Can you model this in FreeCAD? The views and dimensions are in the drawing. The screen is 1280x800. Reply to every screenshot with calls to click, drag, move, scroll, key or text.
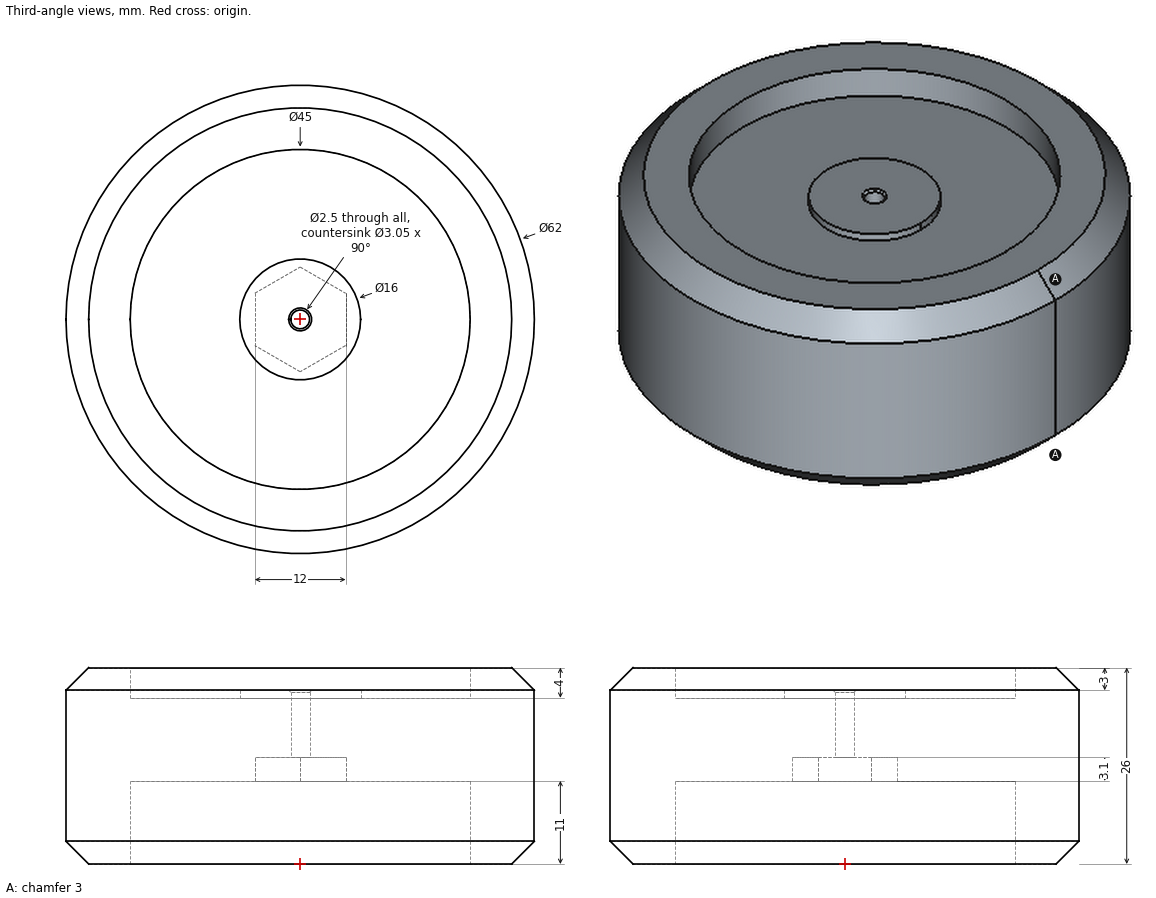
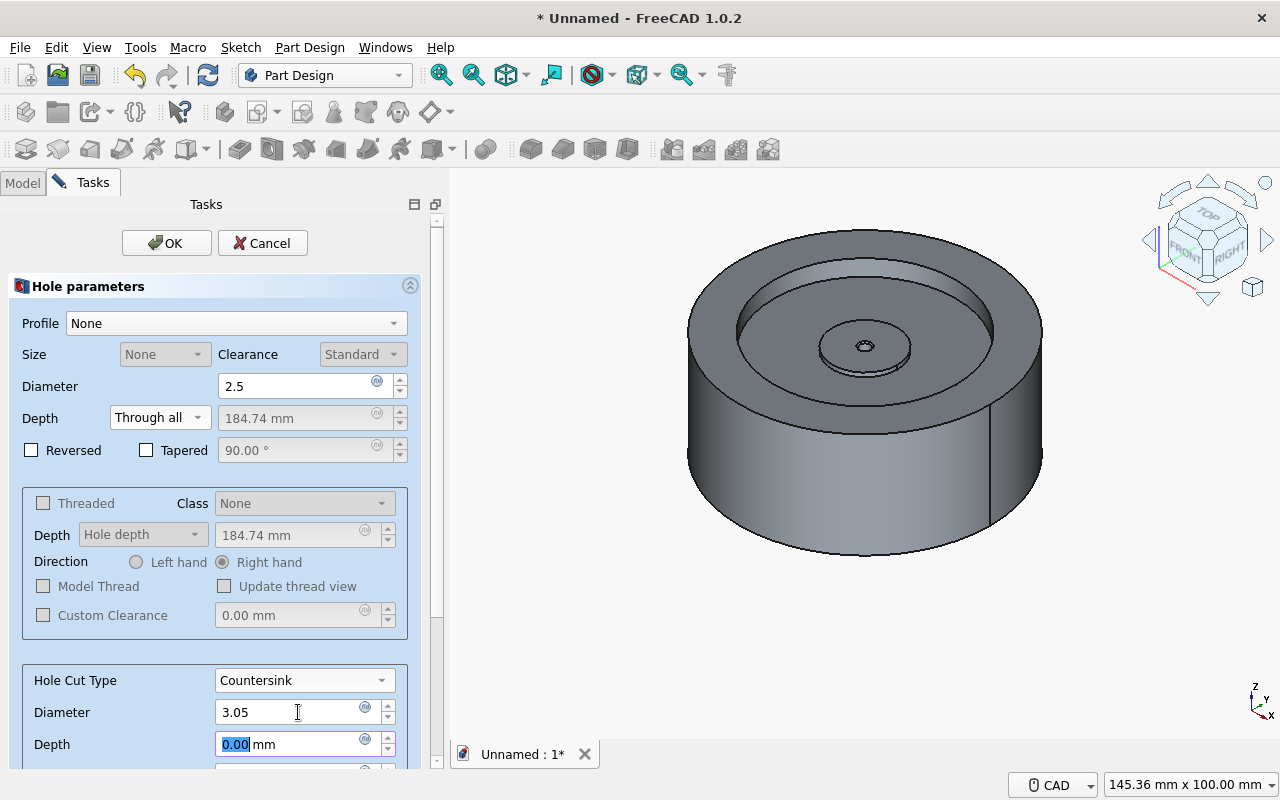
click(167, 243)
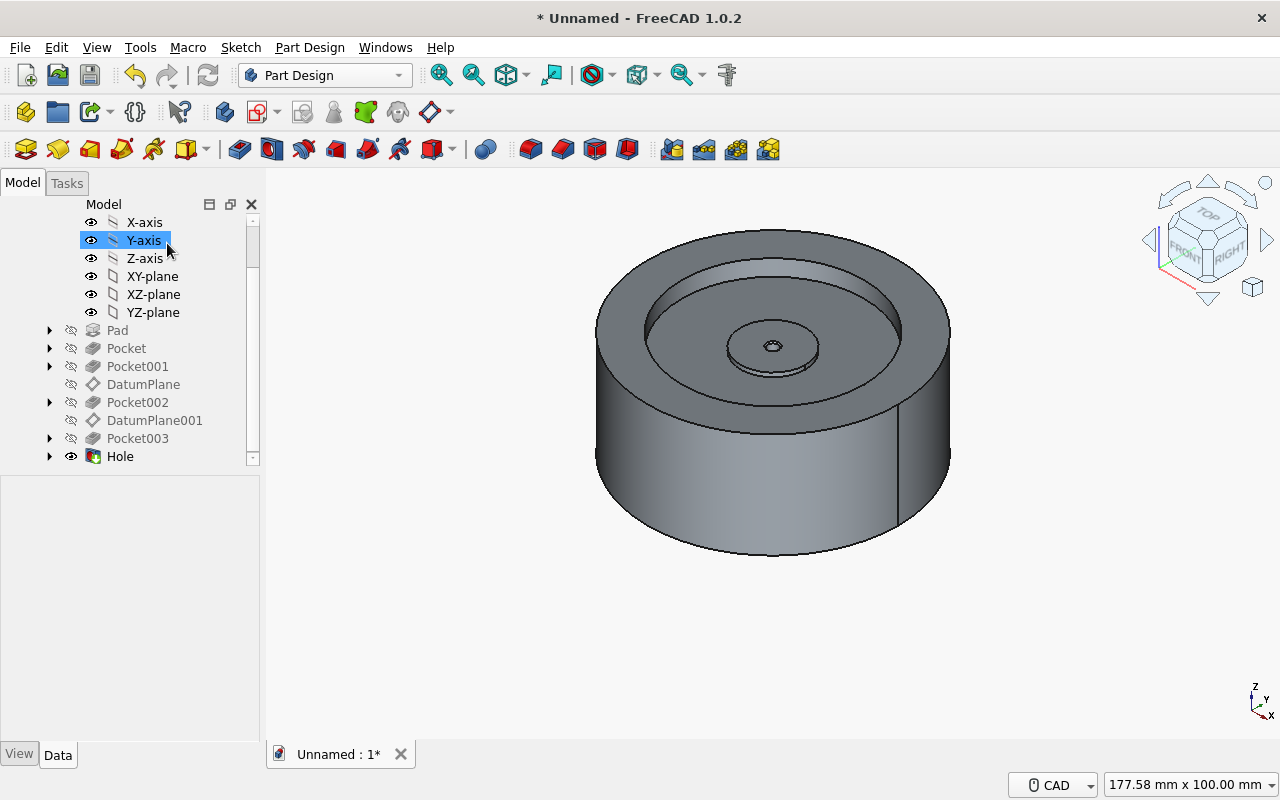
click(693, 544)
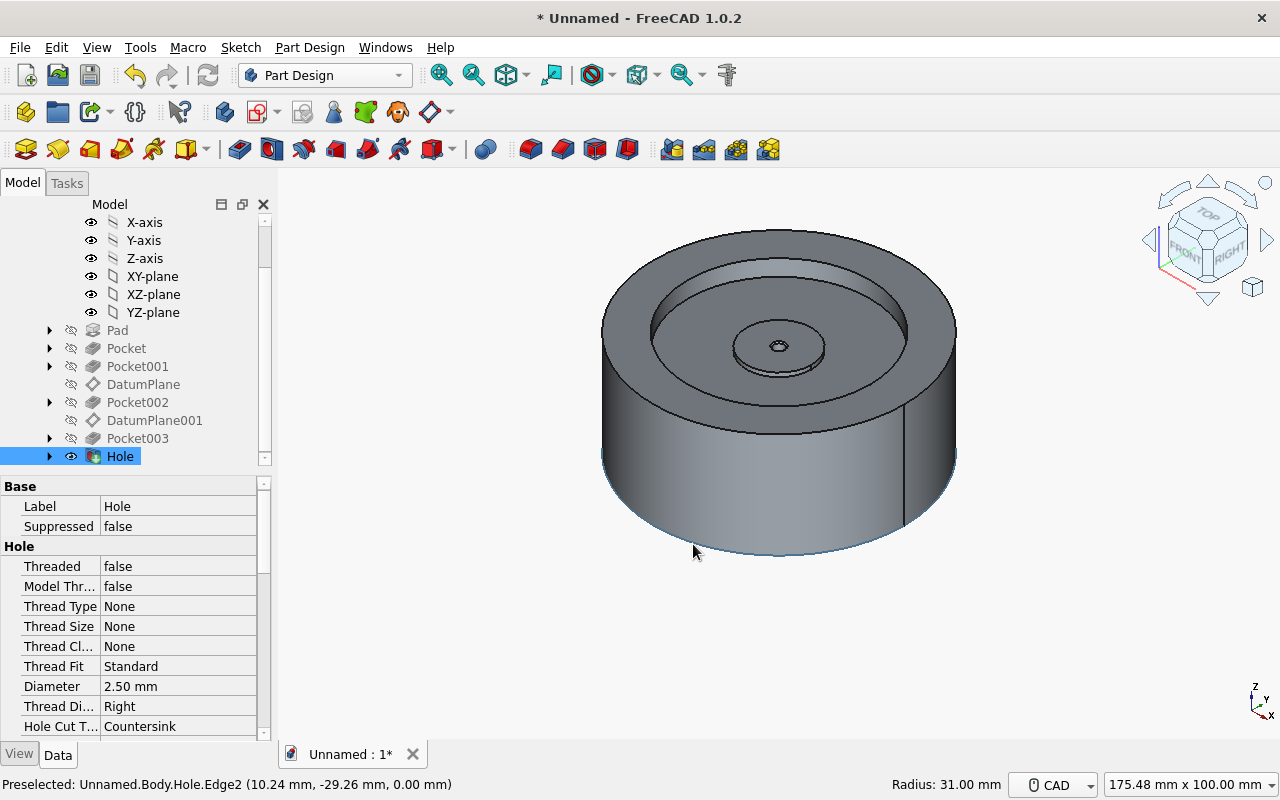
click(621, 378, ctrl)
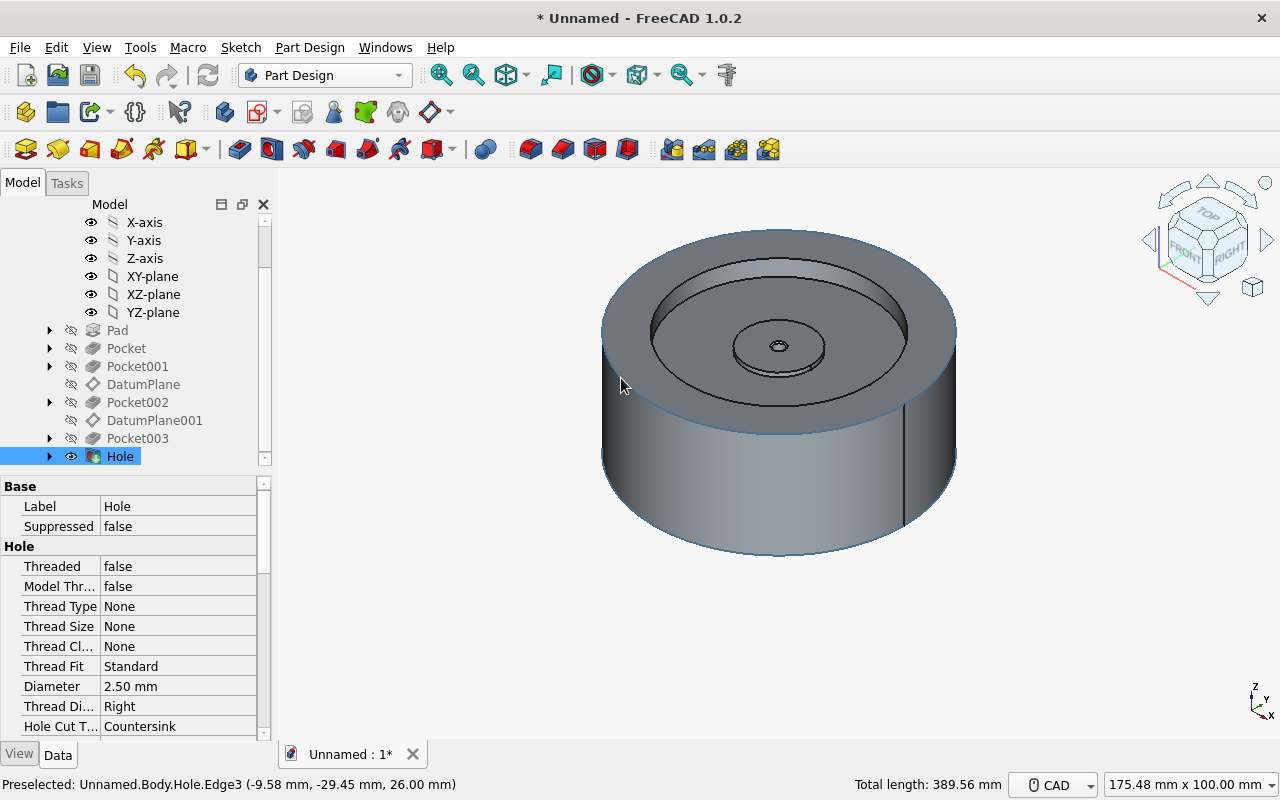
click(564, 150)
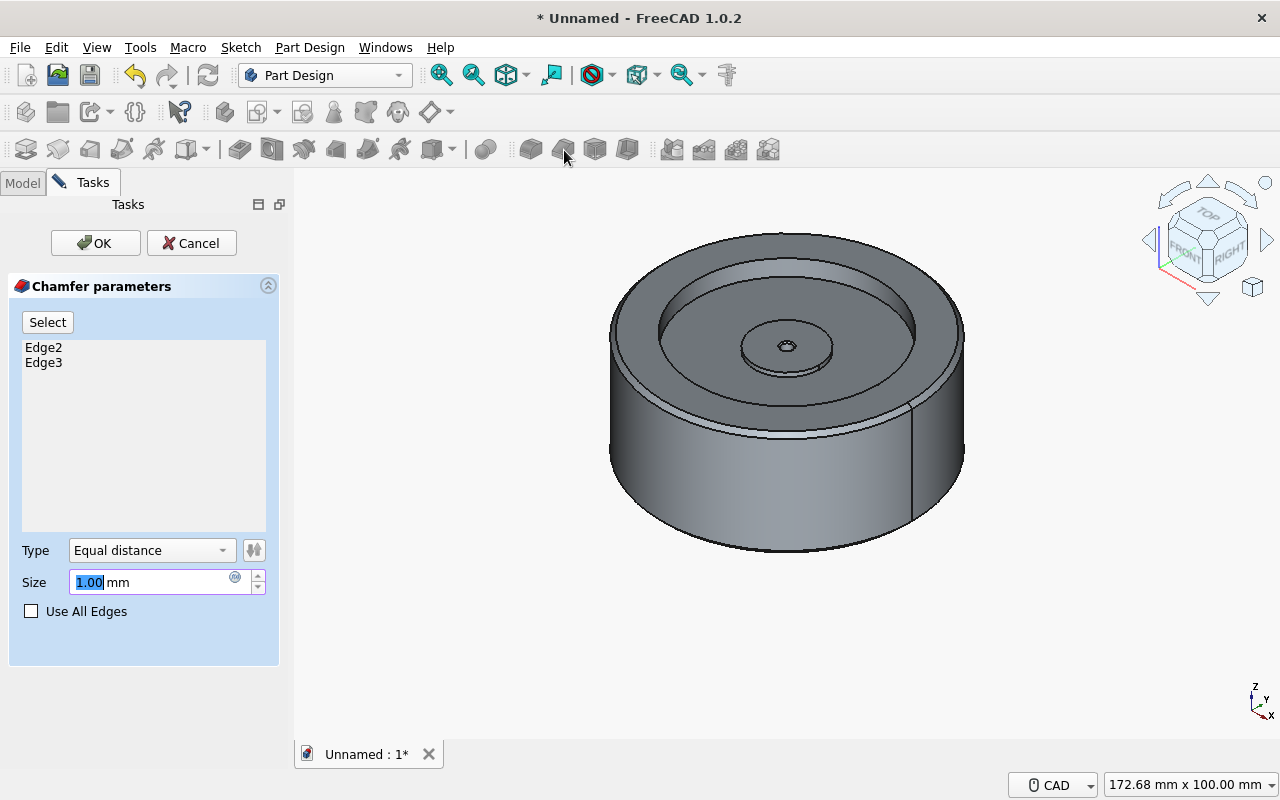
text(3)
key(Tab)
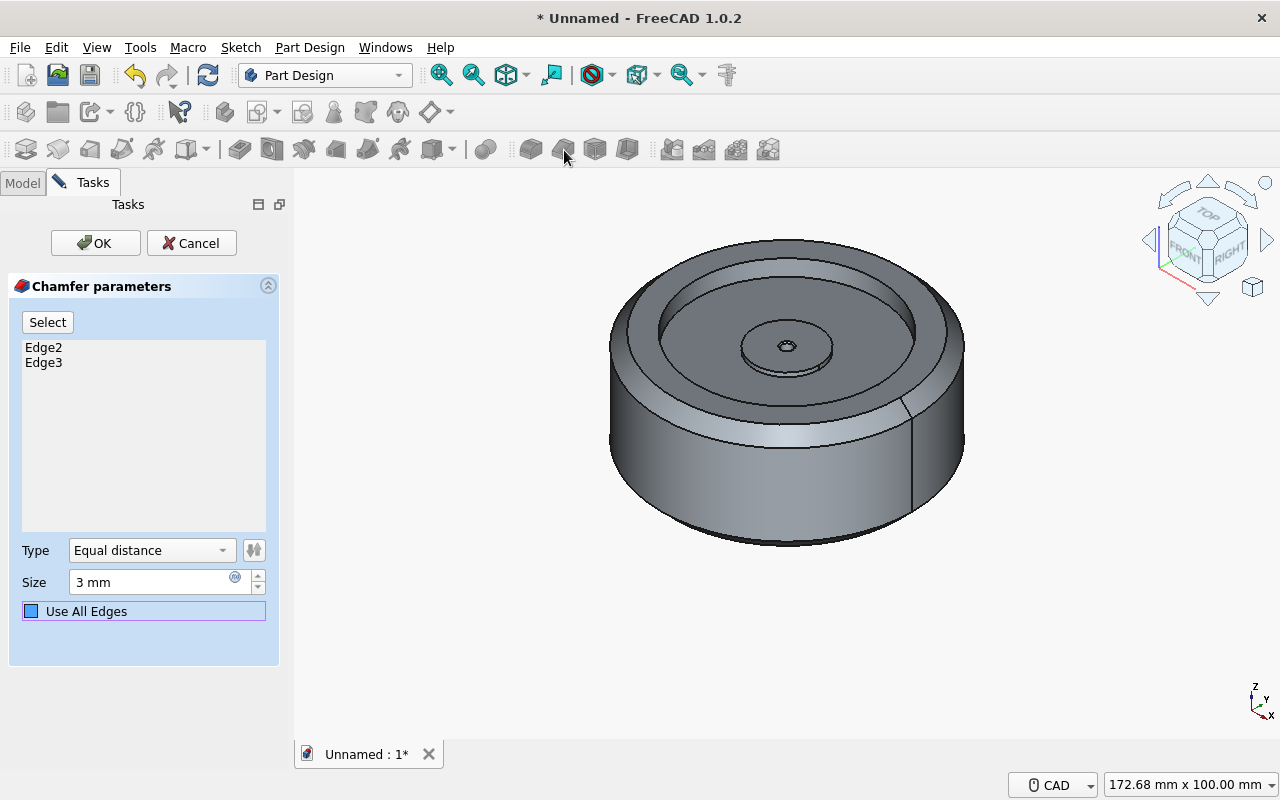
click(96, 243)